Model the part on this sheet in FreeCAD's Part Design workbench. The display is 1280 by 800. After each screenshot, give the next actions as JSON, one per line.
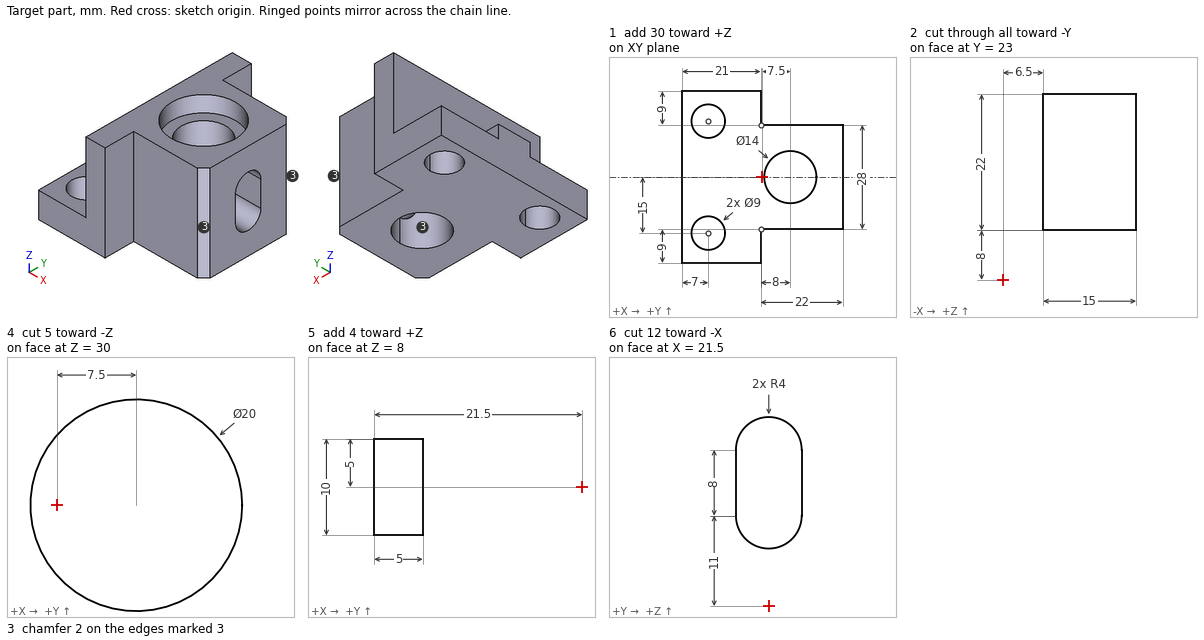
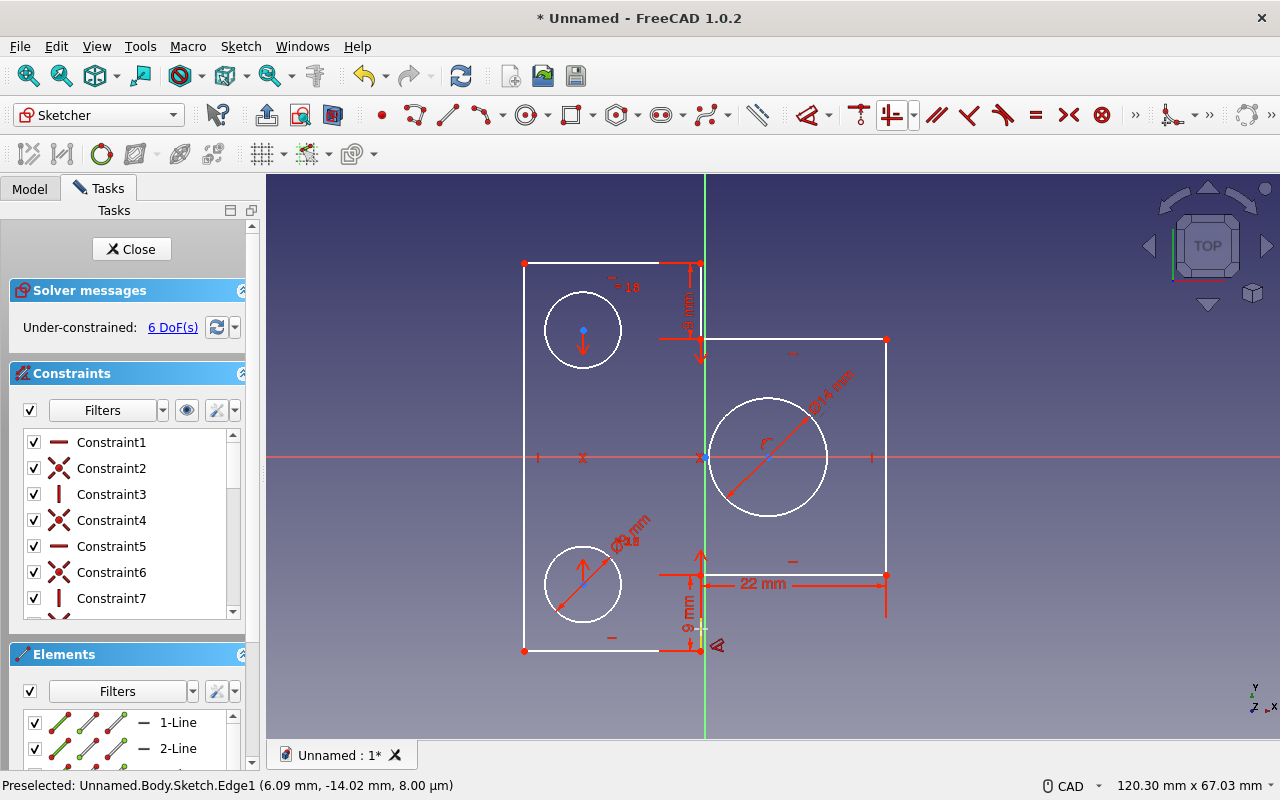
{"action": "left_click", "coordinate": [886, 505]}
{"action": "left_click", "coordinate": [920, 403]}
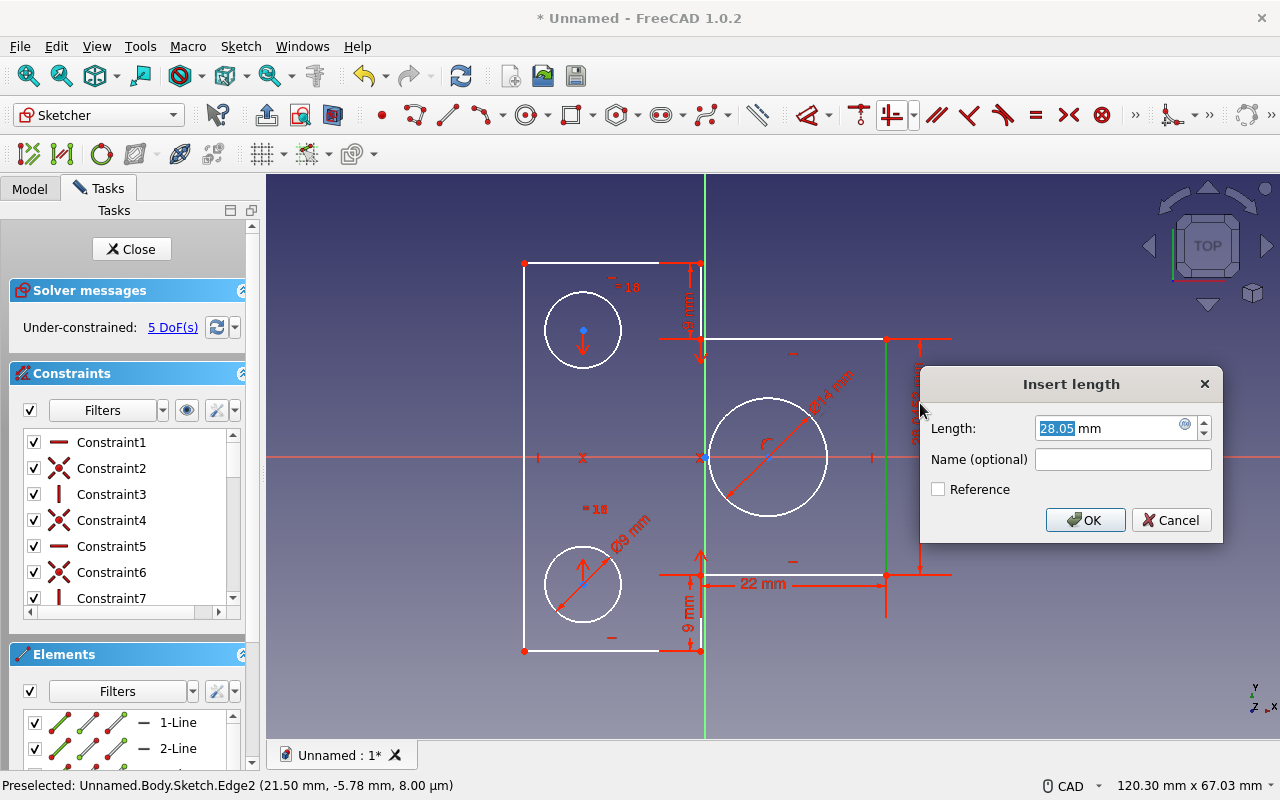
{"action": "type", "text": "28"}
{"action": "key", "text": "Return"}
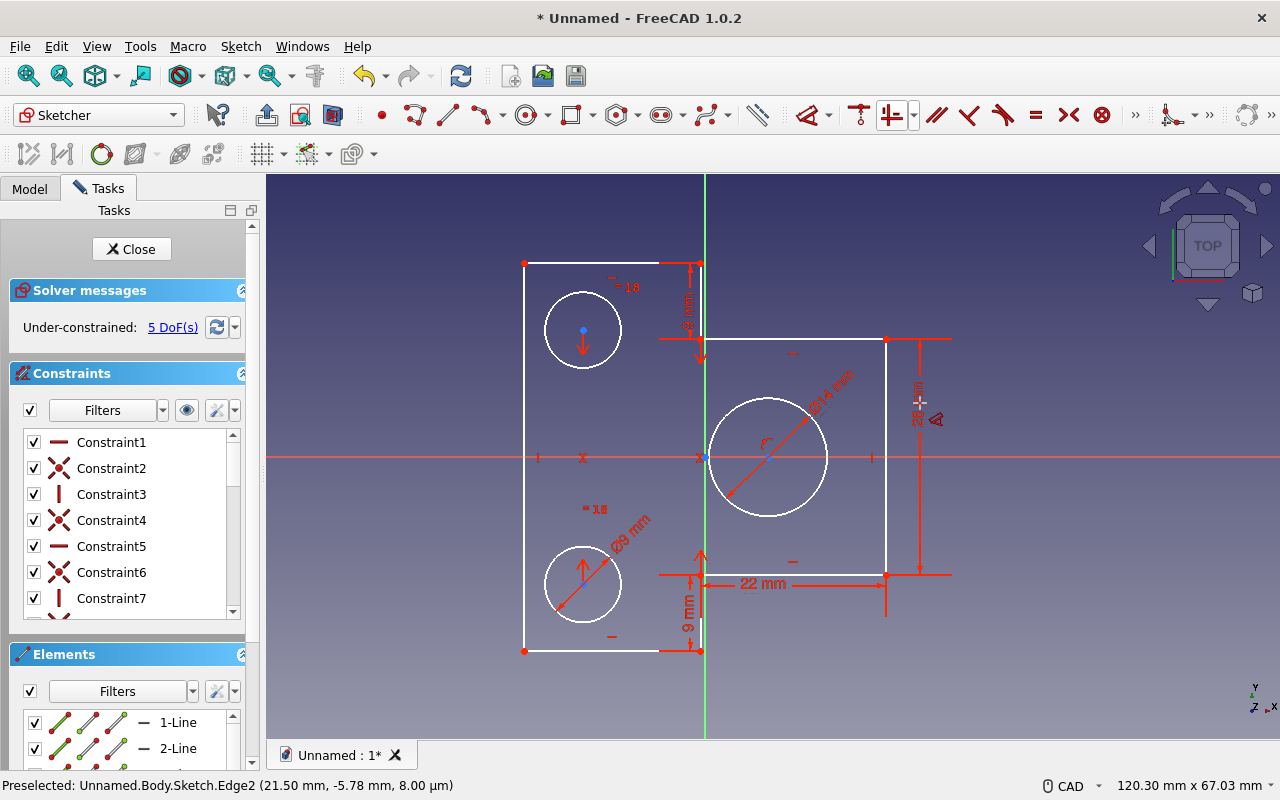
{"action": "left_click", "coordinate": [648, 263]}
{"action": "left_click", "coordinate": [612, 229]}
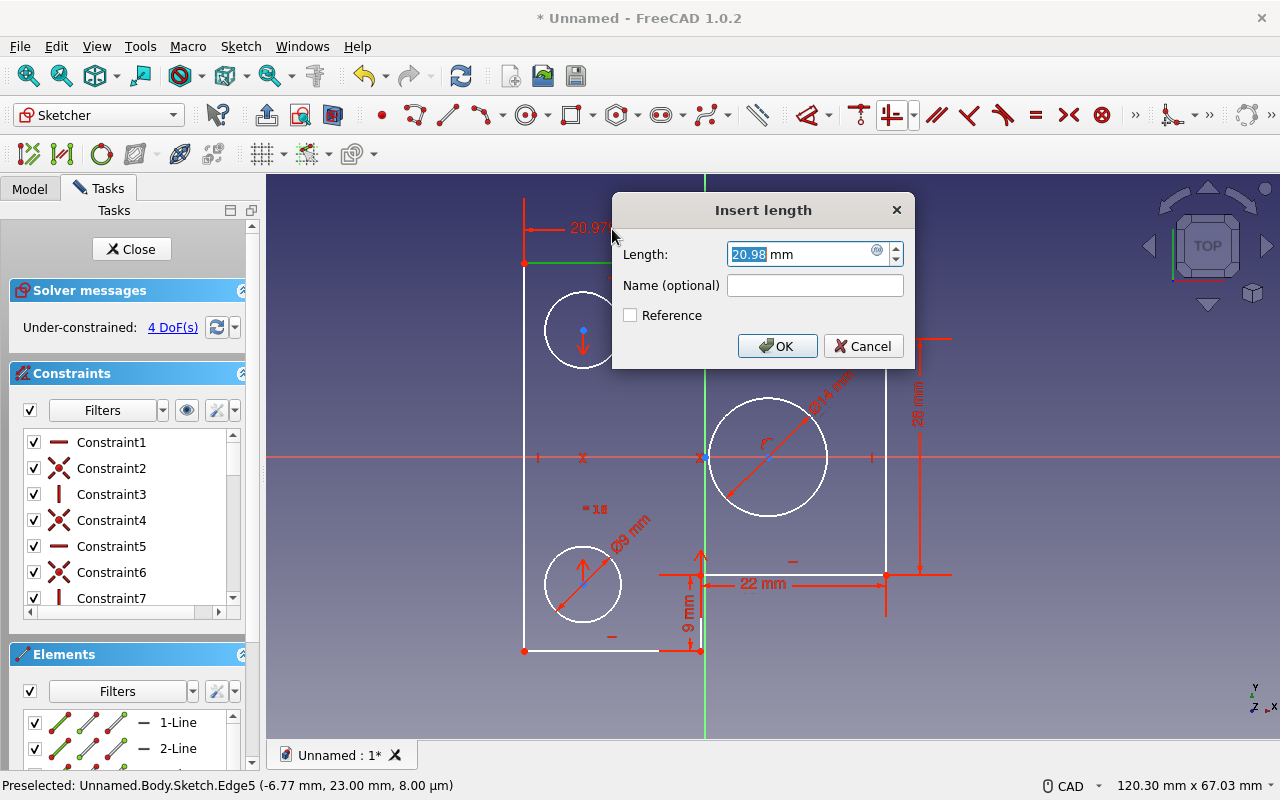
{"action": "type", "text": "21"}
{"action": "key", "text": "Return"}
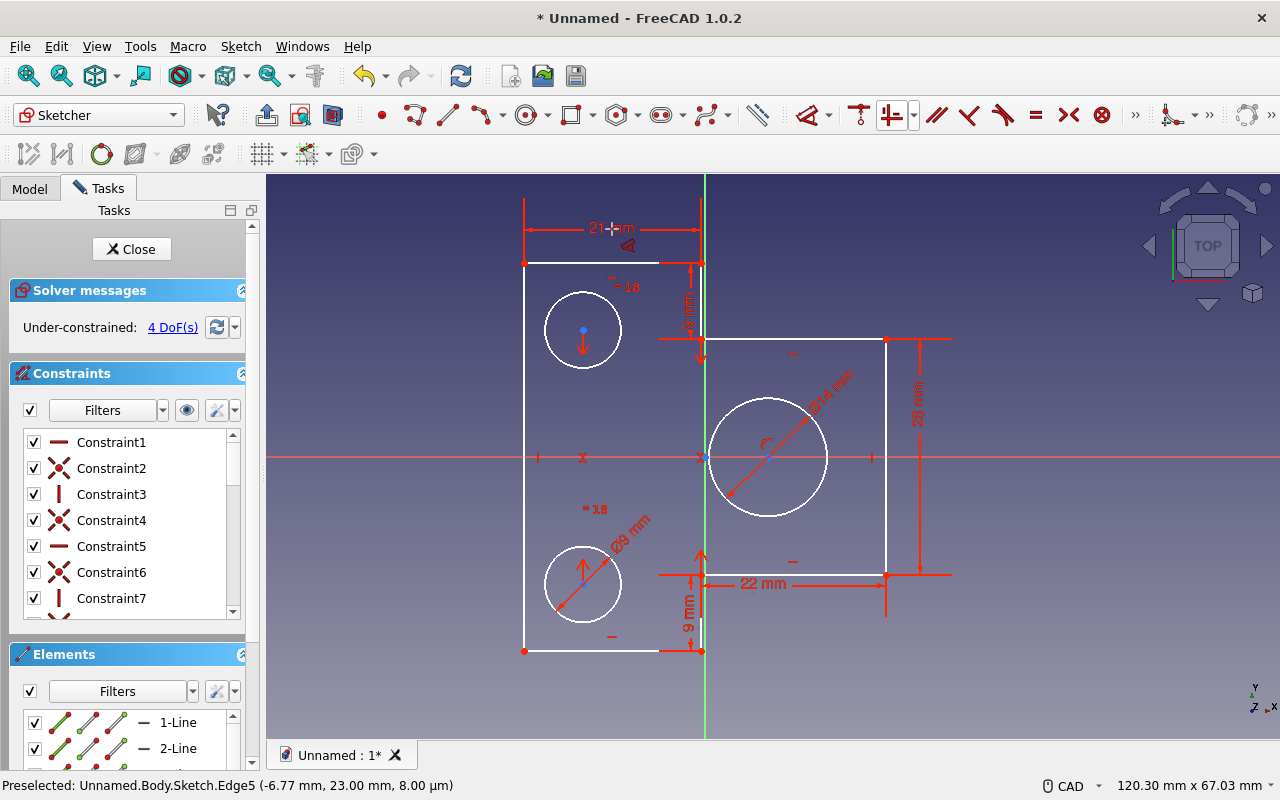
{"action": "left_click", "coordinate": [583, 584]}
{"action": "left_click", "coordinate": [549, 521]}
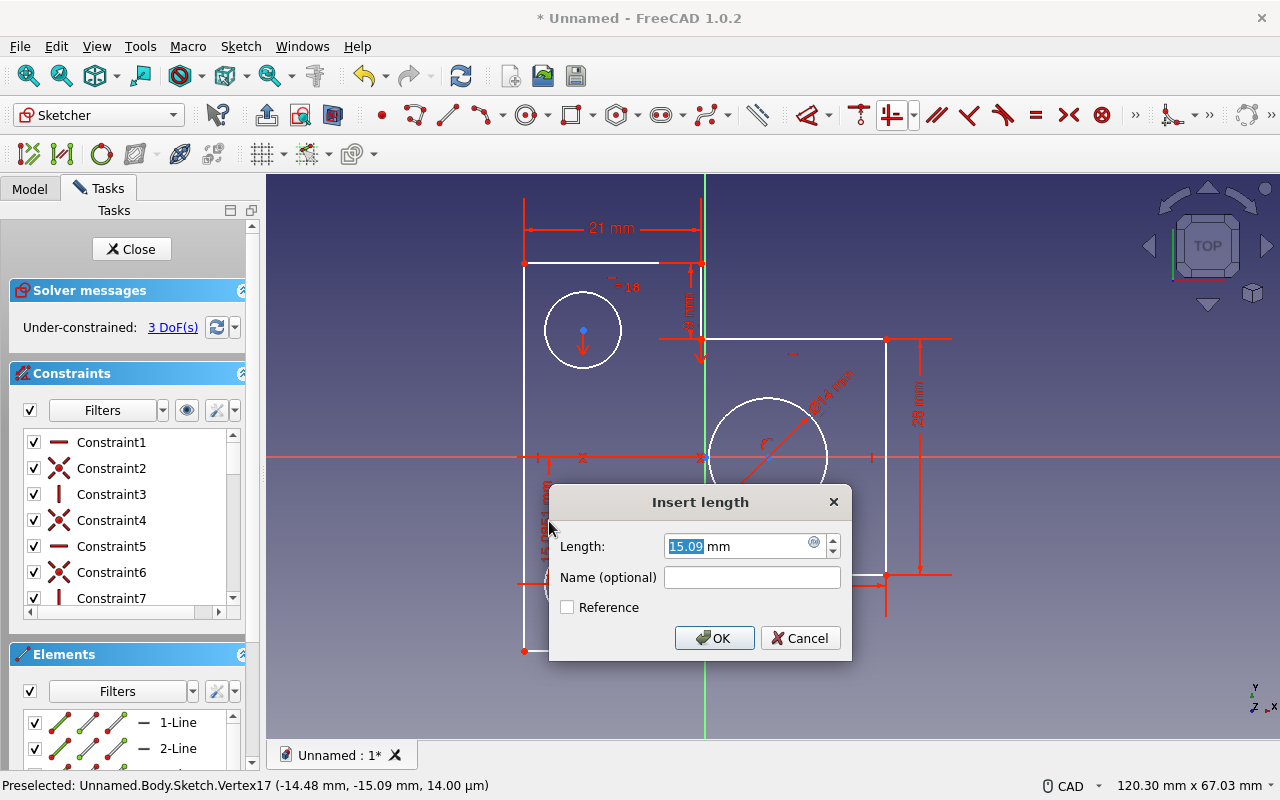
{"action": "type", "text": "15"}
{"action": "key", "text": "Return"}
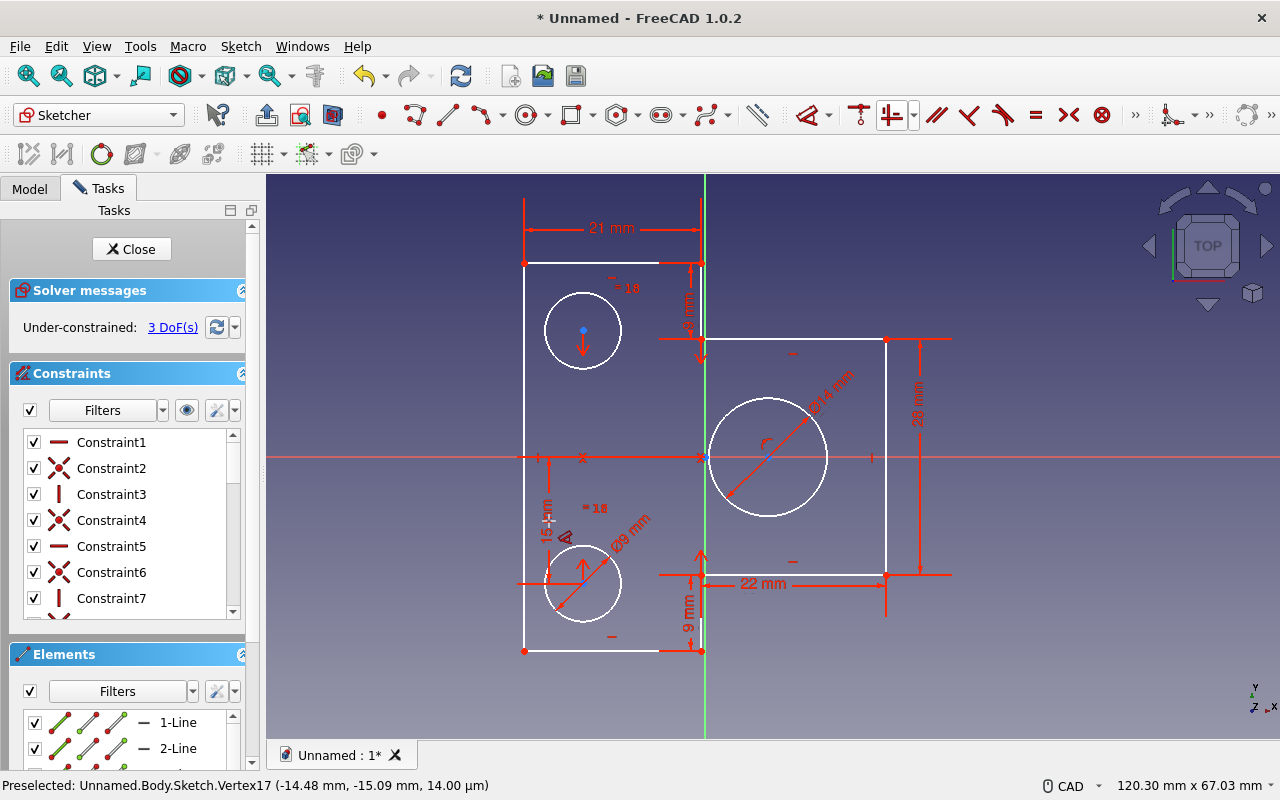
{"action": "left_click", "coordinate": [524, 651]}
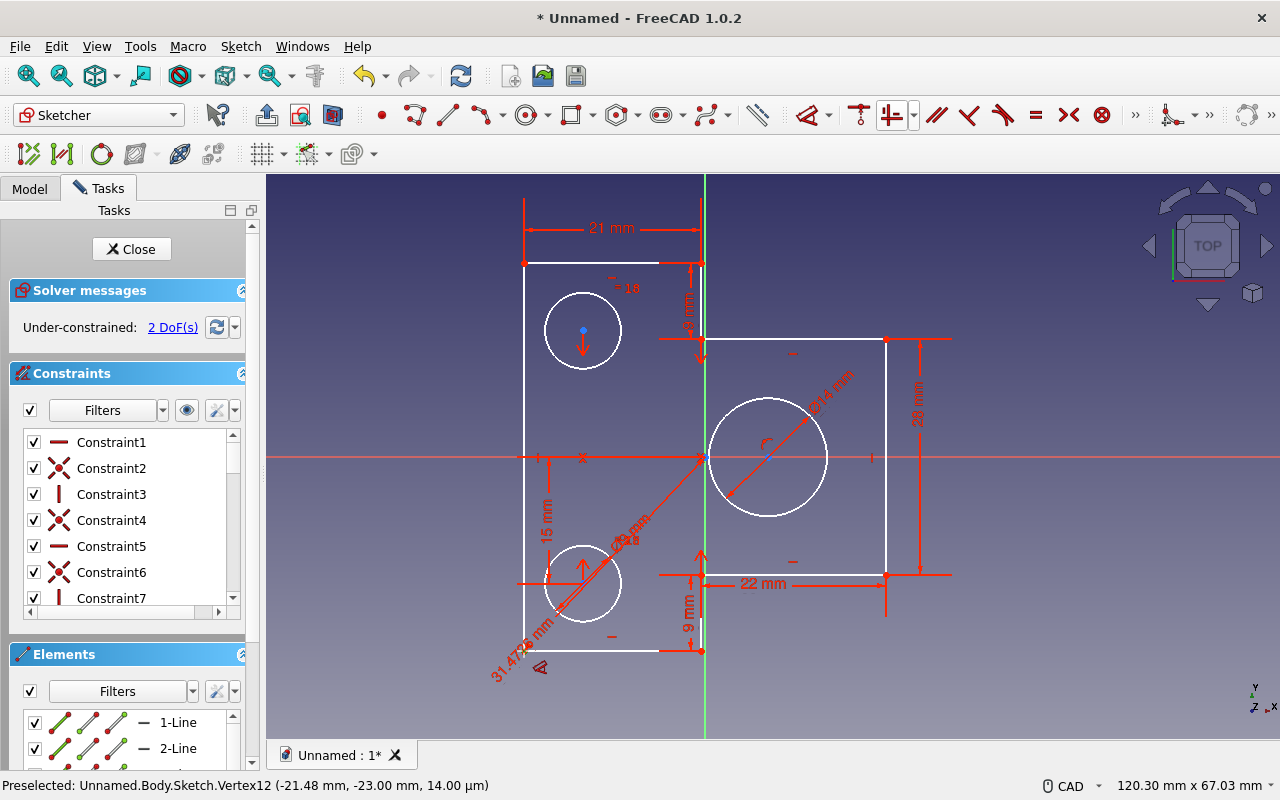
{"action": "left_click", "coordinate": [583, 584]}
{"action": "left_click", "coordinate": [554, 685]}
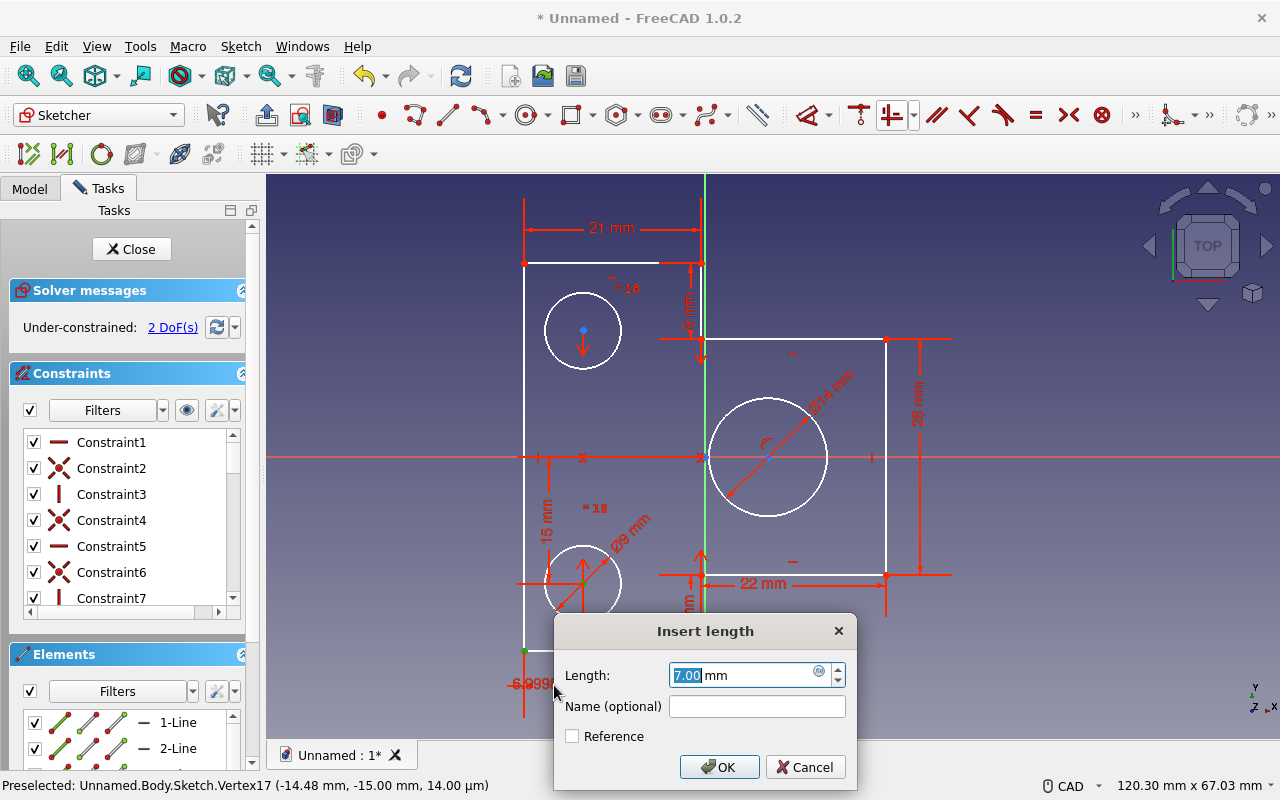
{"action": "type", "text": "7"}
{"action": "key", "text": "Return"}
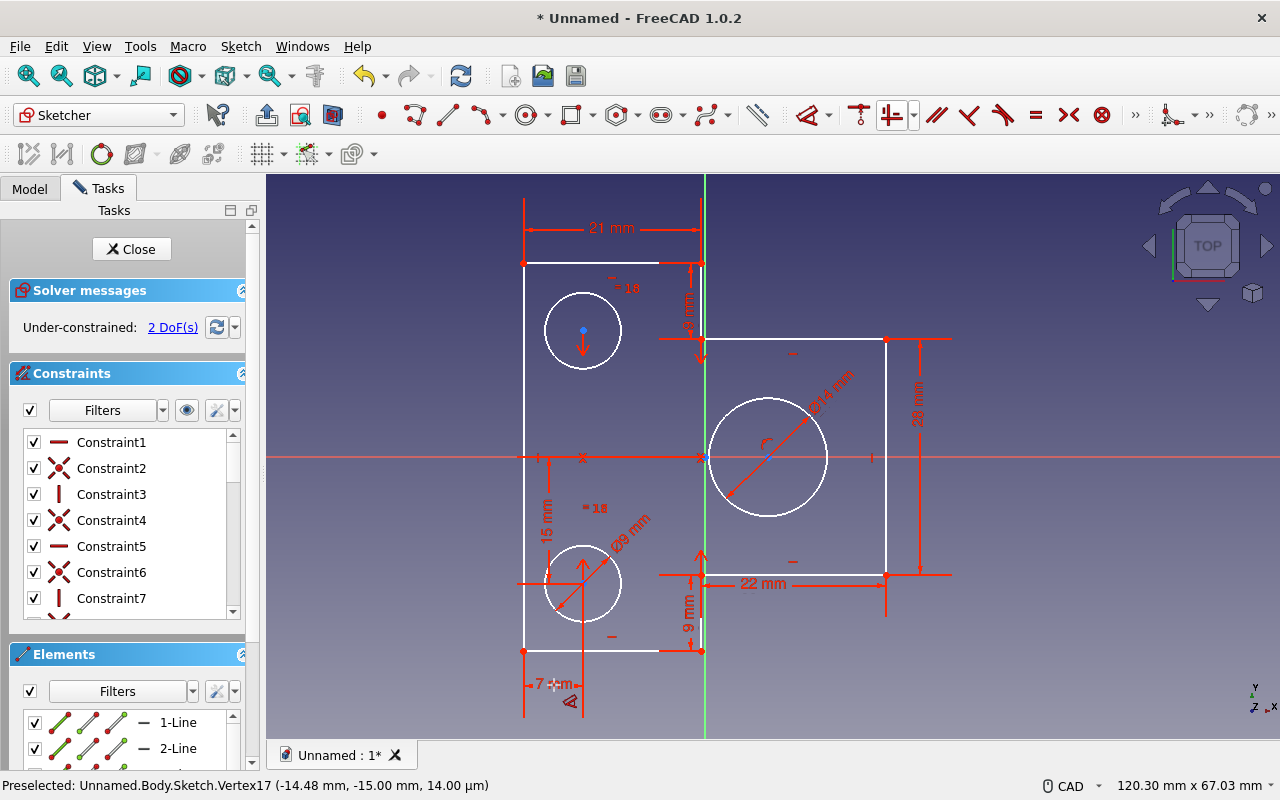
{"action": "left_click", "coordinate": [701, 575]}